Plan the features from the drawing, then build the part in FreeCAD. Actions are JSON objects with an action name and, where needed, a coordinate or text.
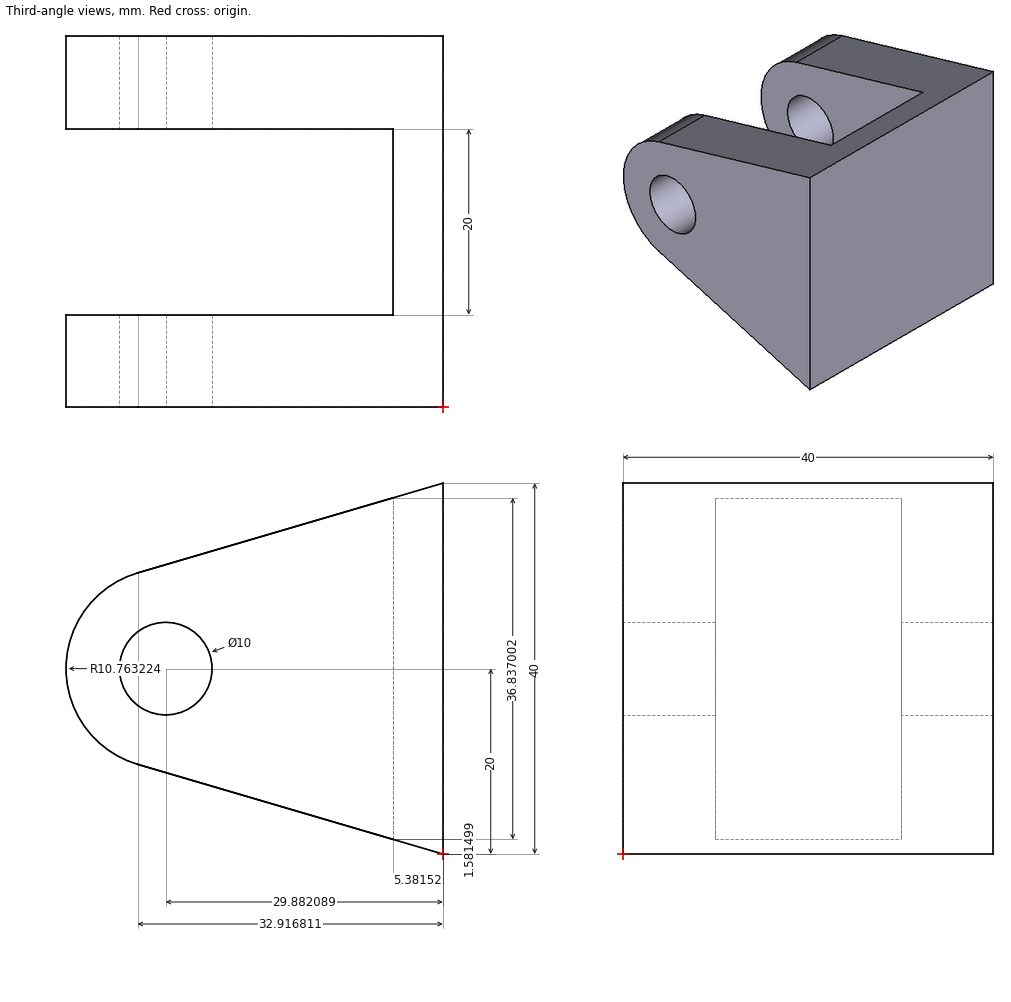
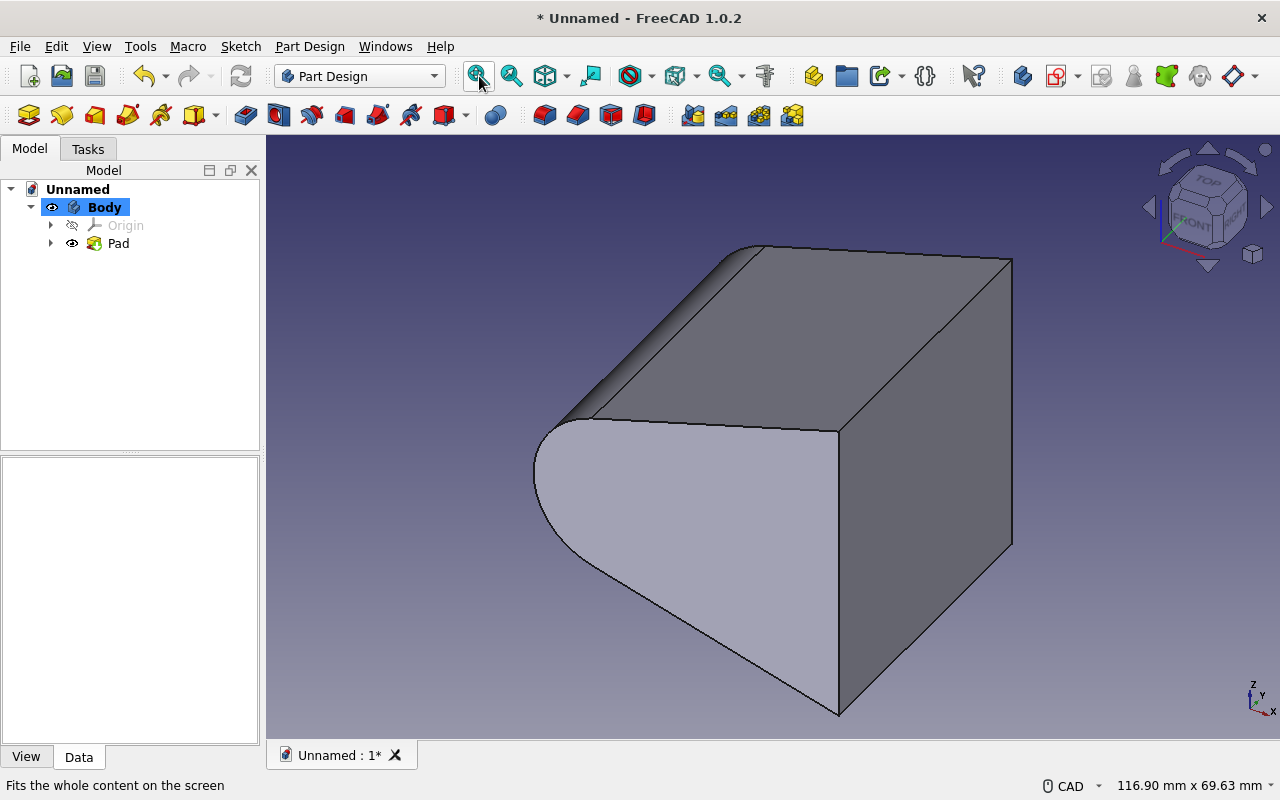
{"action": "left_click", "coordinate": [51, 225]}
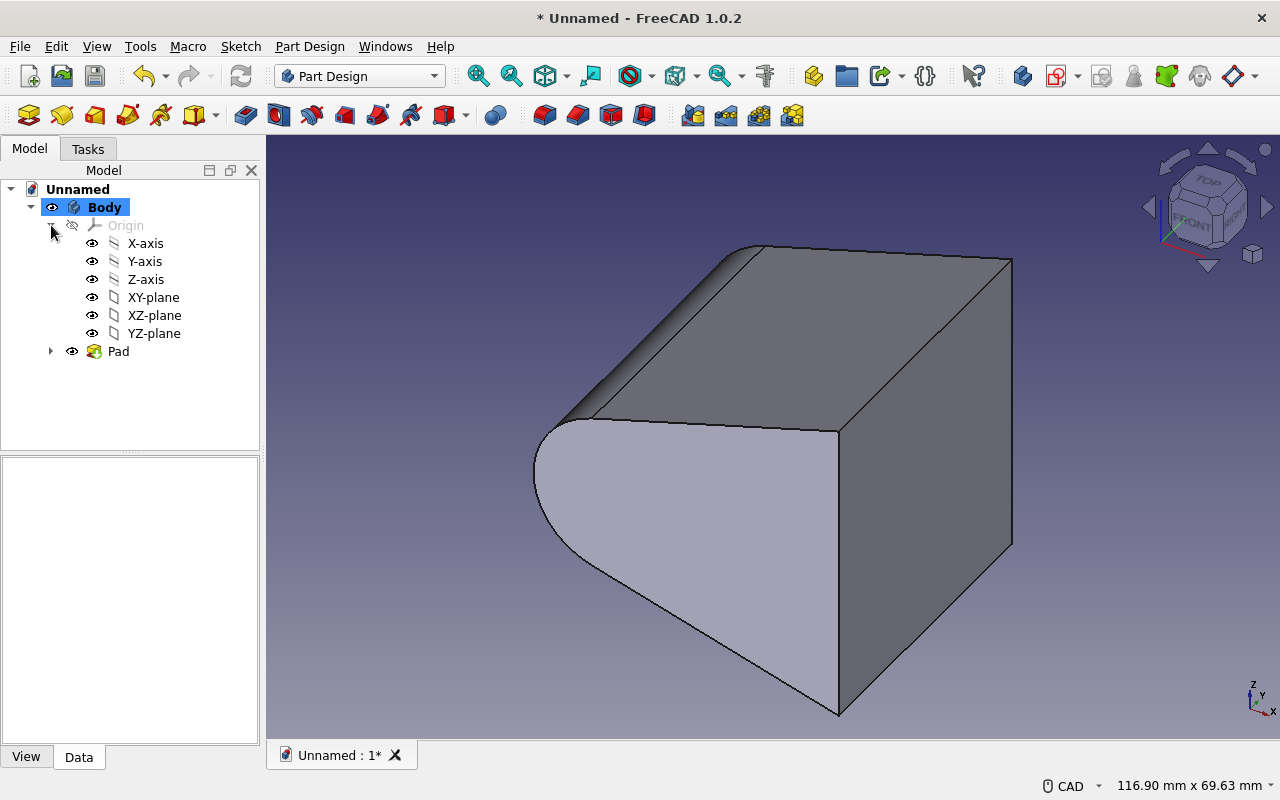
{"action": "left_click", "coordinate": [137, 315]}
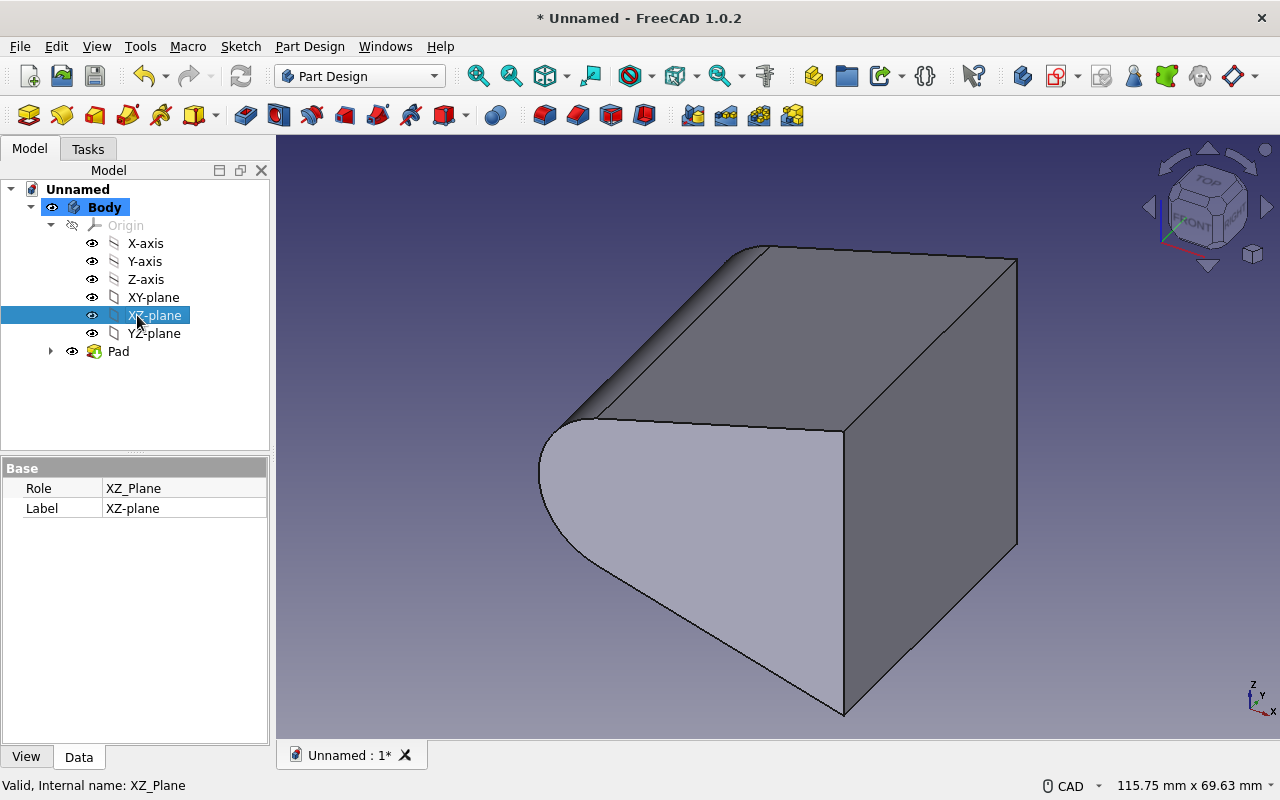
{"action": "left_click", "coordinate": [1232, 76]}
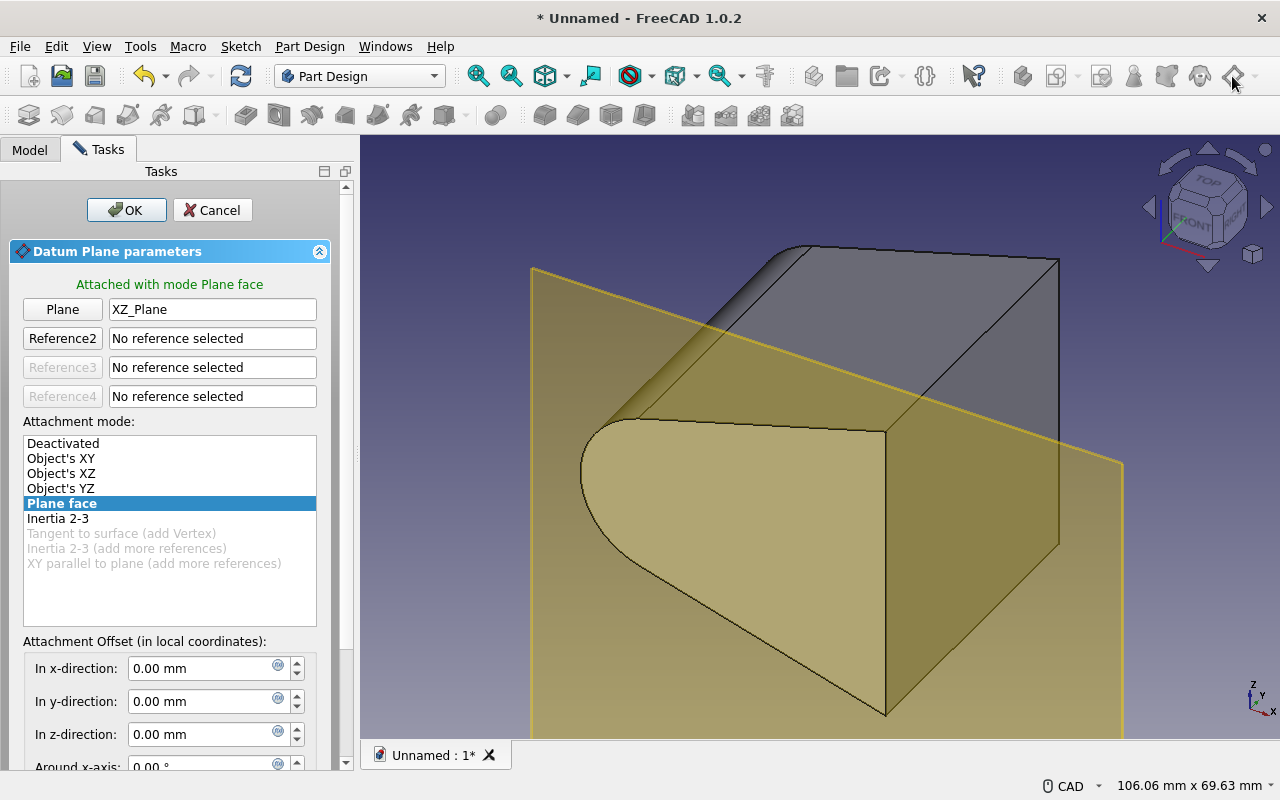
{"action": "triple_click", "coordinate": [210, 734]}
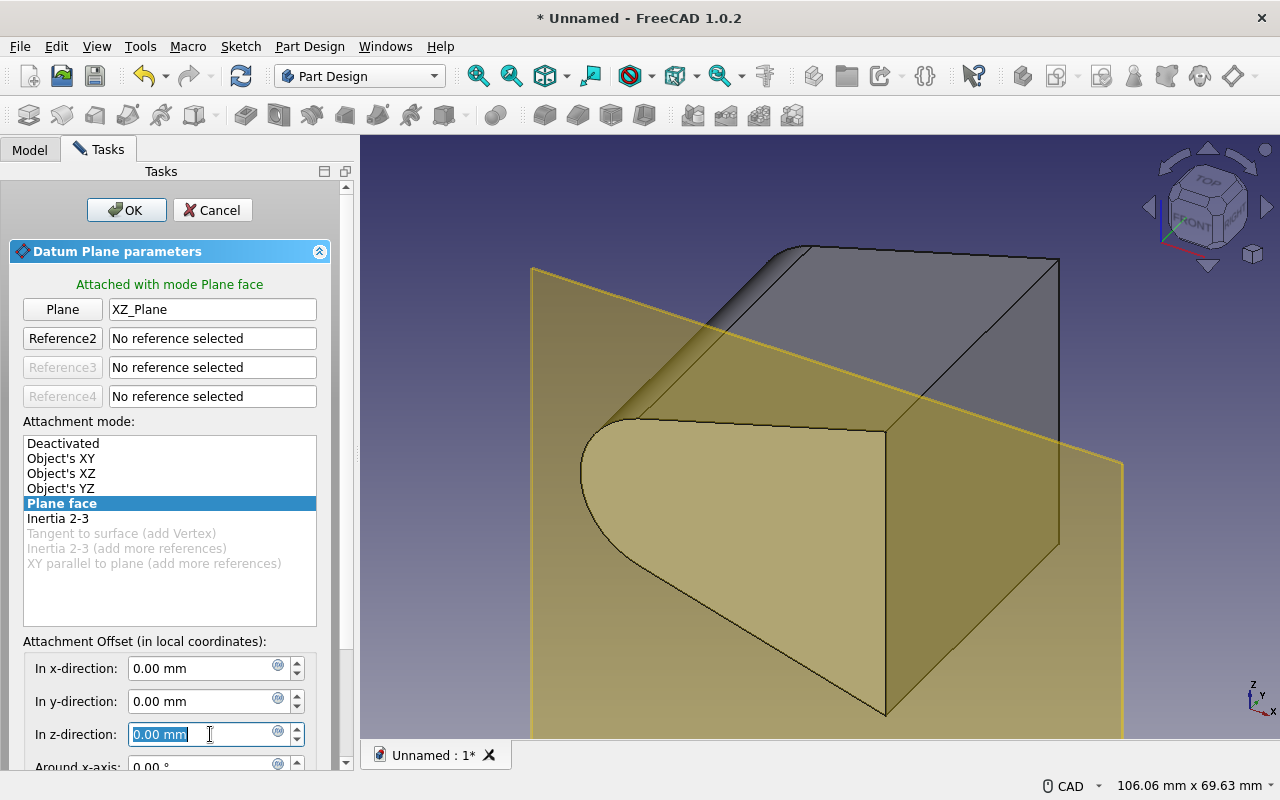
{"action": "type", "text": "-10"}
{"action": "key", "text": "Tab"}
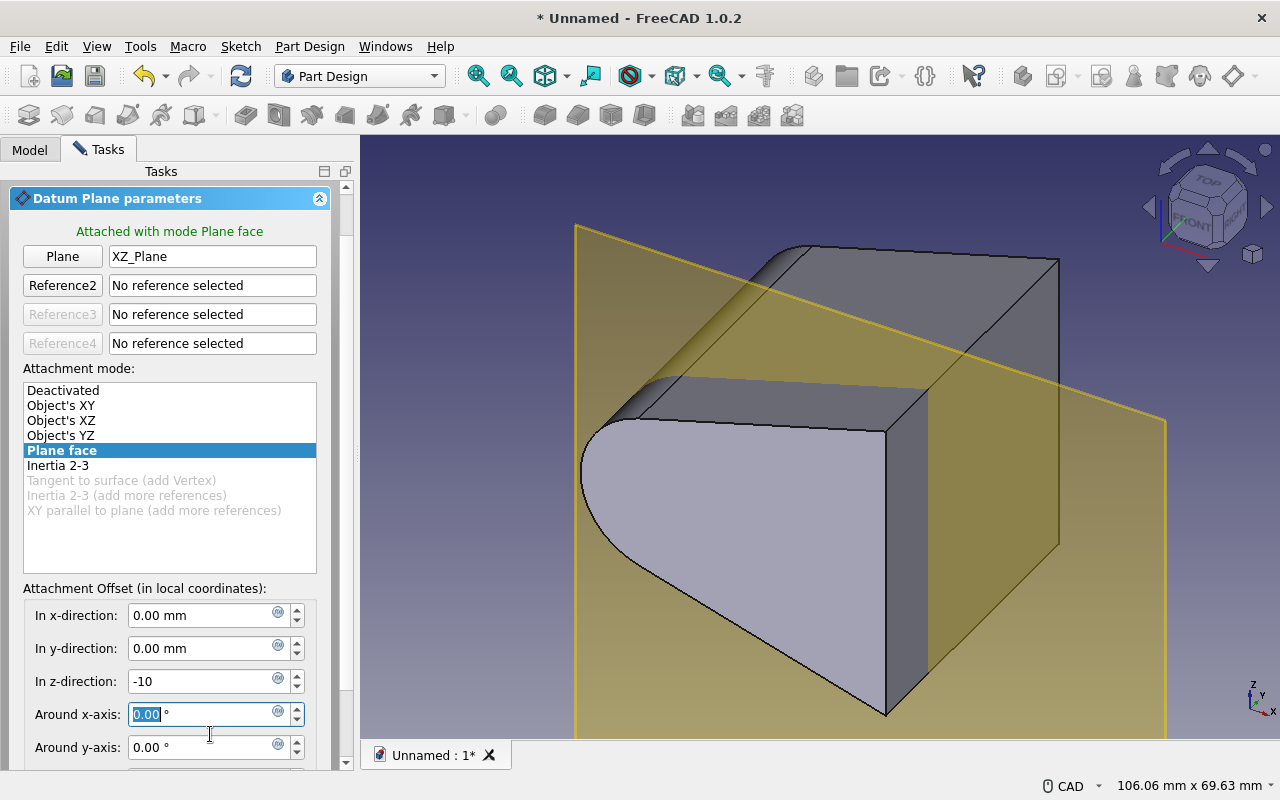
{"action": "scroll", "coordinate": [346, 476], "scroll_direction": "up", "scroll_amount": 2}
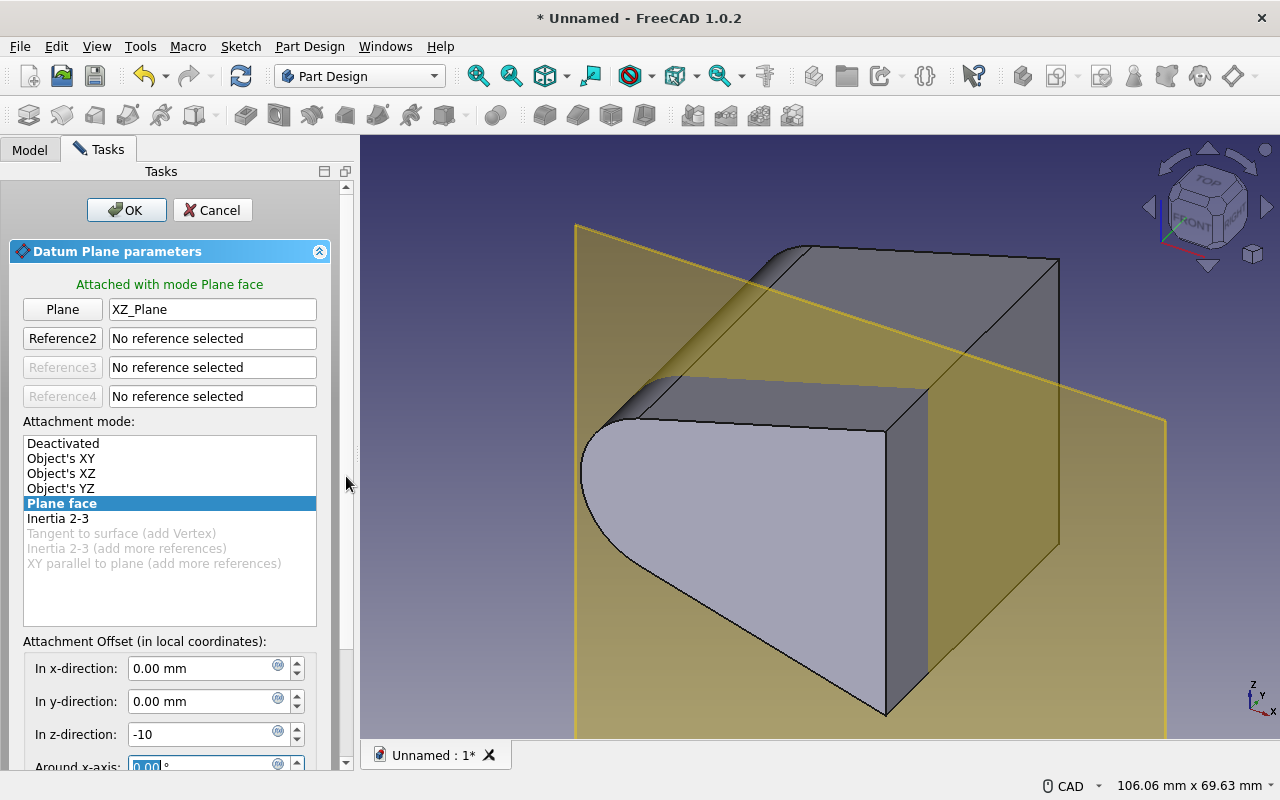
{"action": "left_click", "coordinate": [127, 210]}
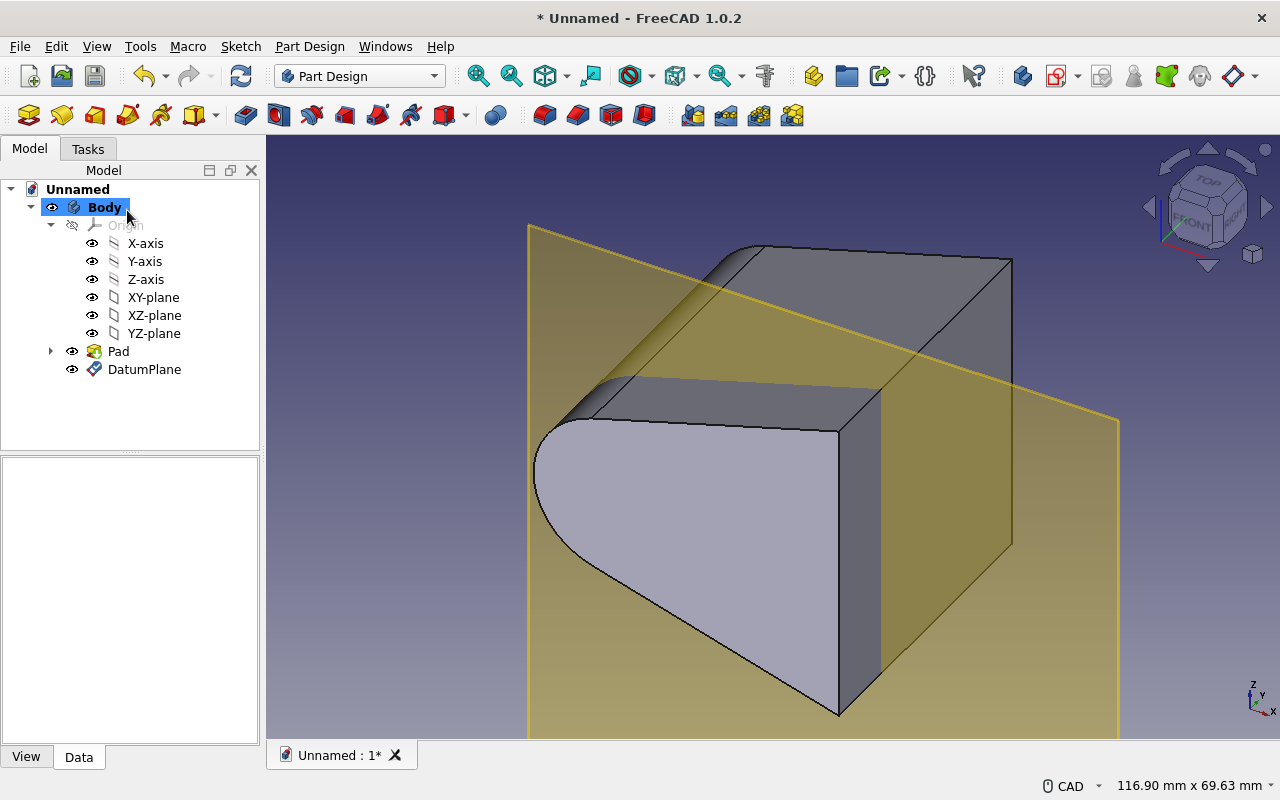
{"action": "left_click", "coordinate": [117, 369]}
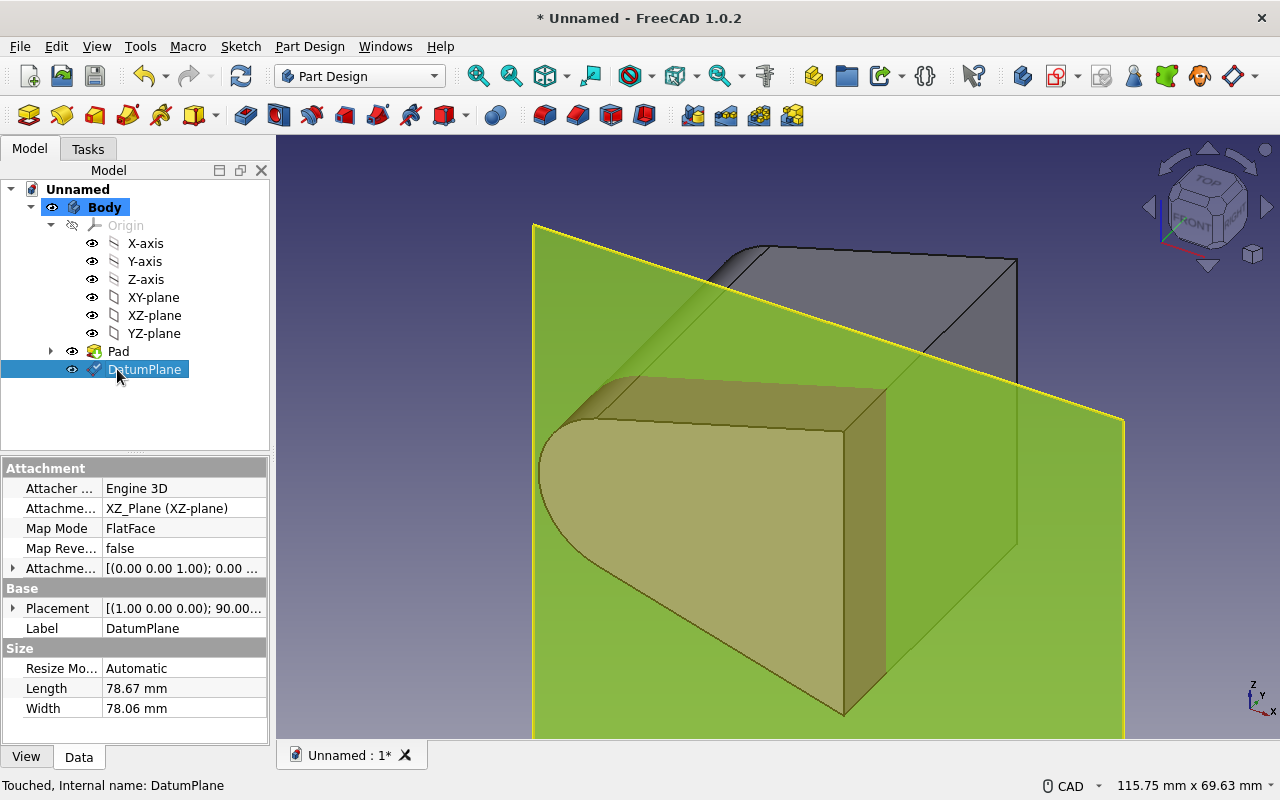
{"action": "left_click", "coordinate": [1056, 76]}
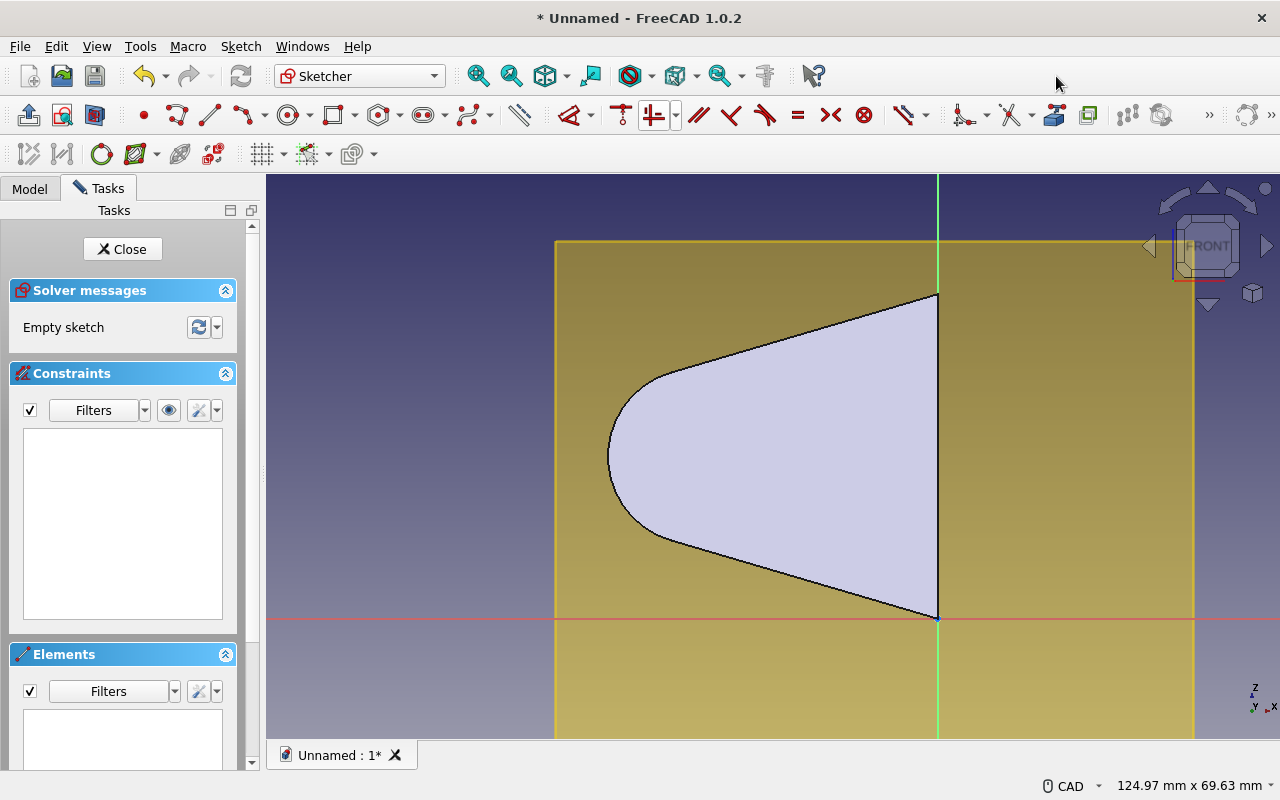
{"action": "left_click", "coordinate": [95, 116]}